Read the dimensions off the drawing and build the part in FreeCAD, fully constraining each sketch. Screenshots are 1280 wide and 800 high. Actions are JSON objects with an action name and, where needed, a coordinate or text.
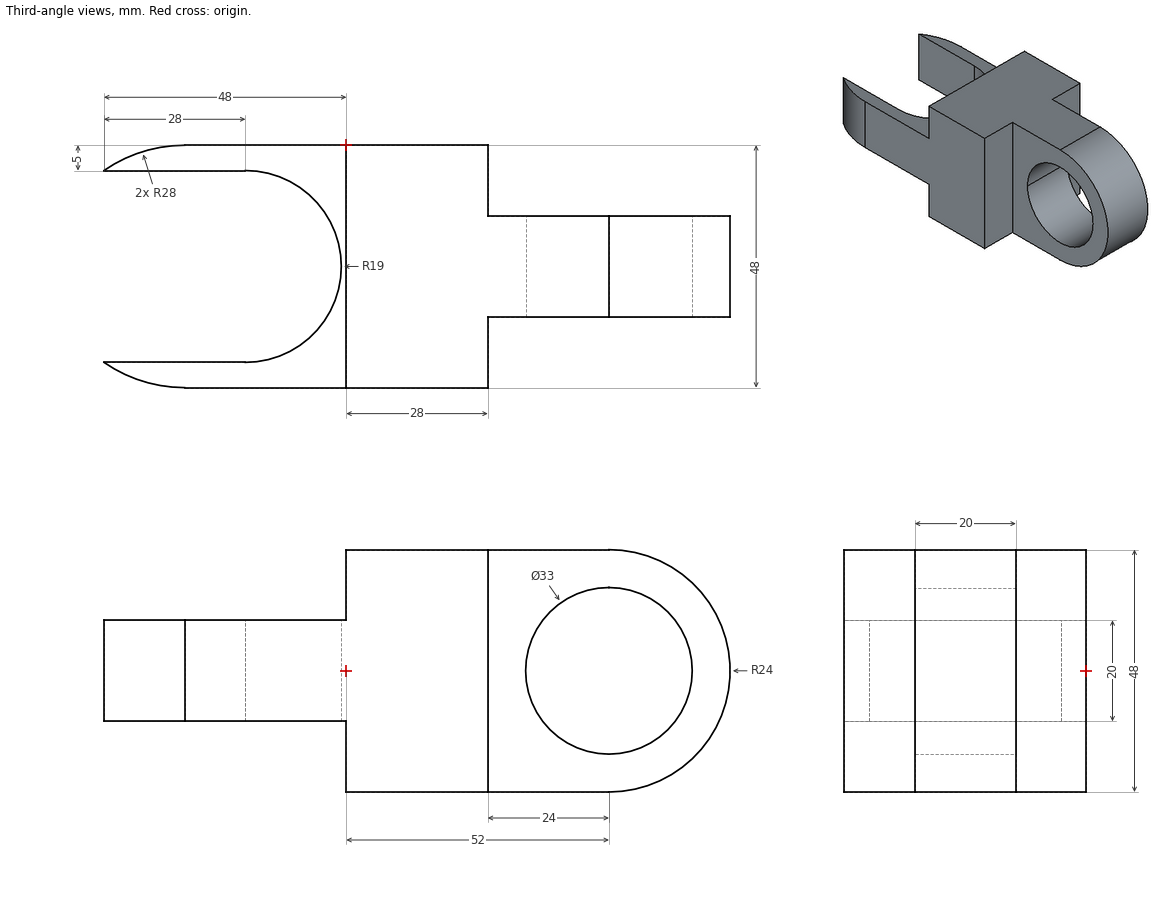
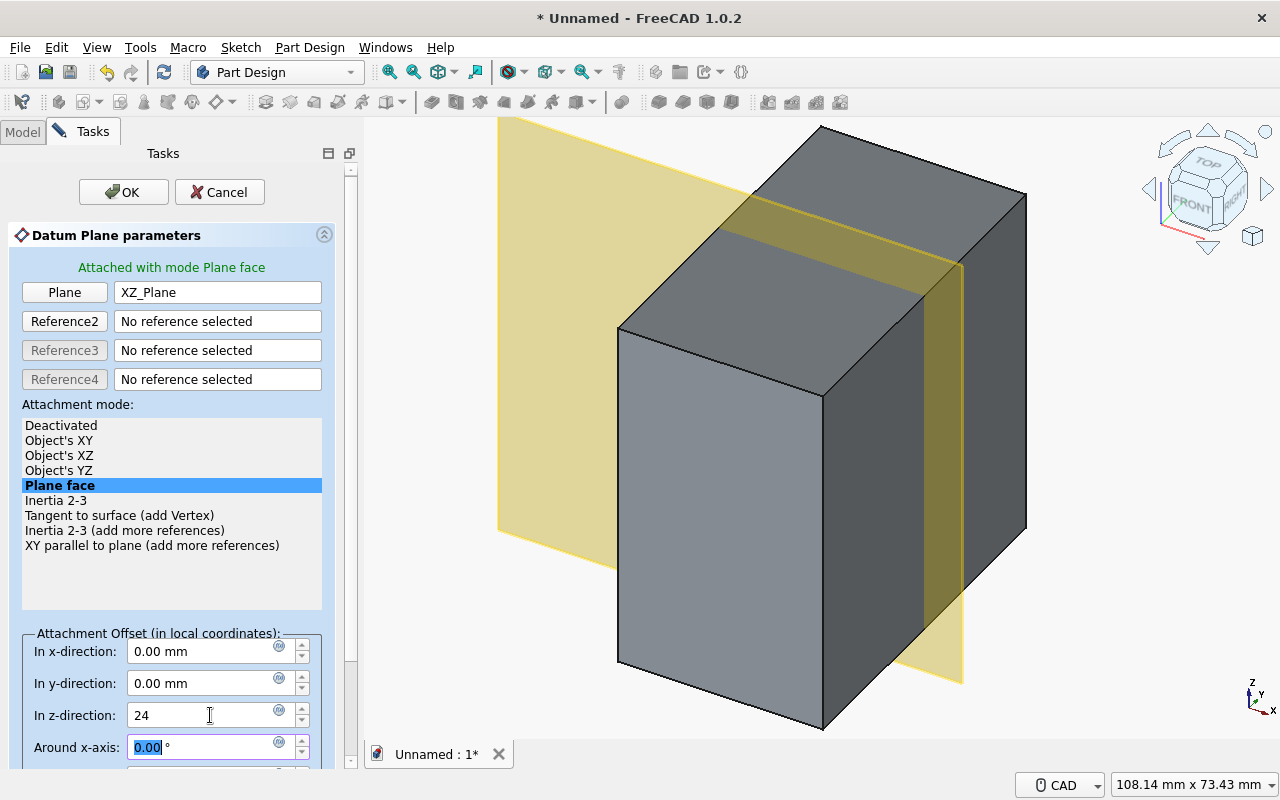
{"action": "left_click", "coordinate": [124, 192]}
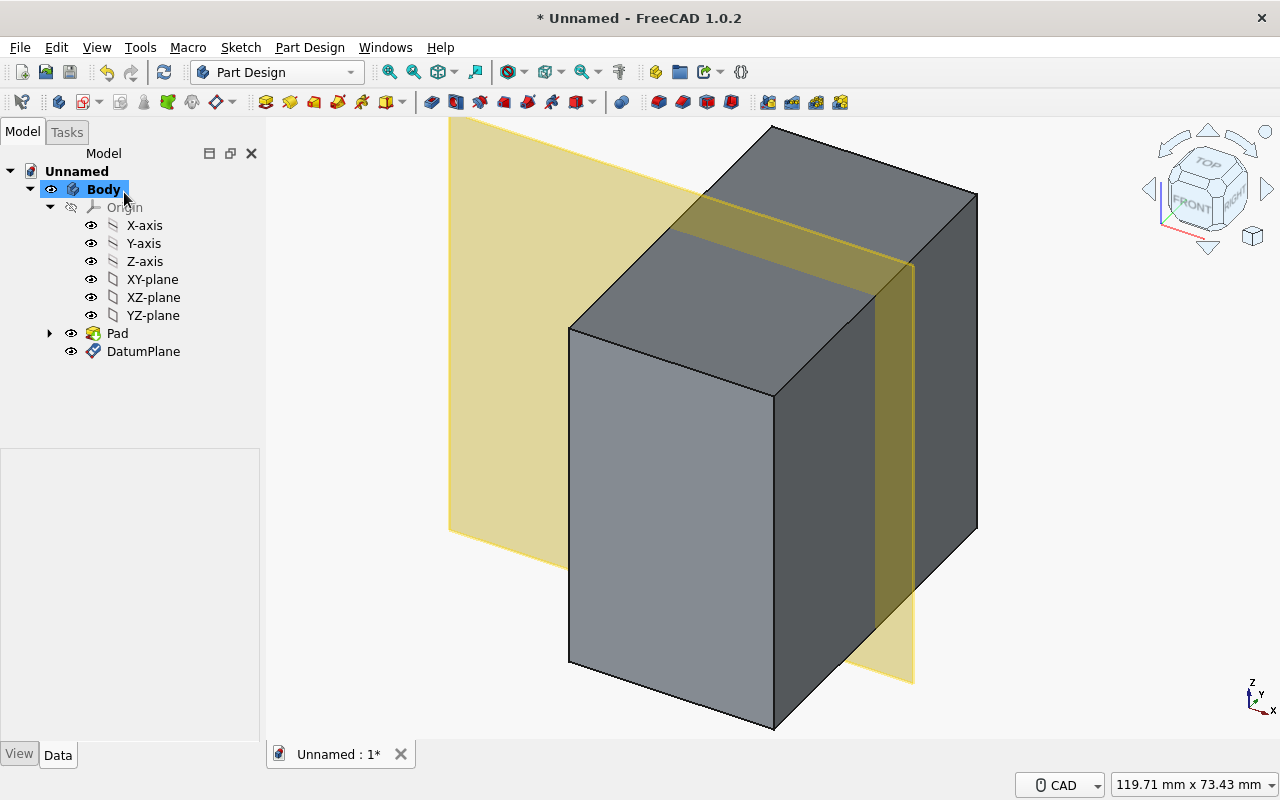
{"action": "left_click", "coordinate": [116, 351]}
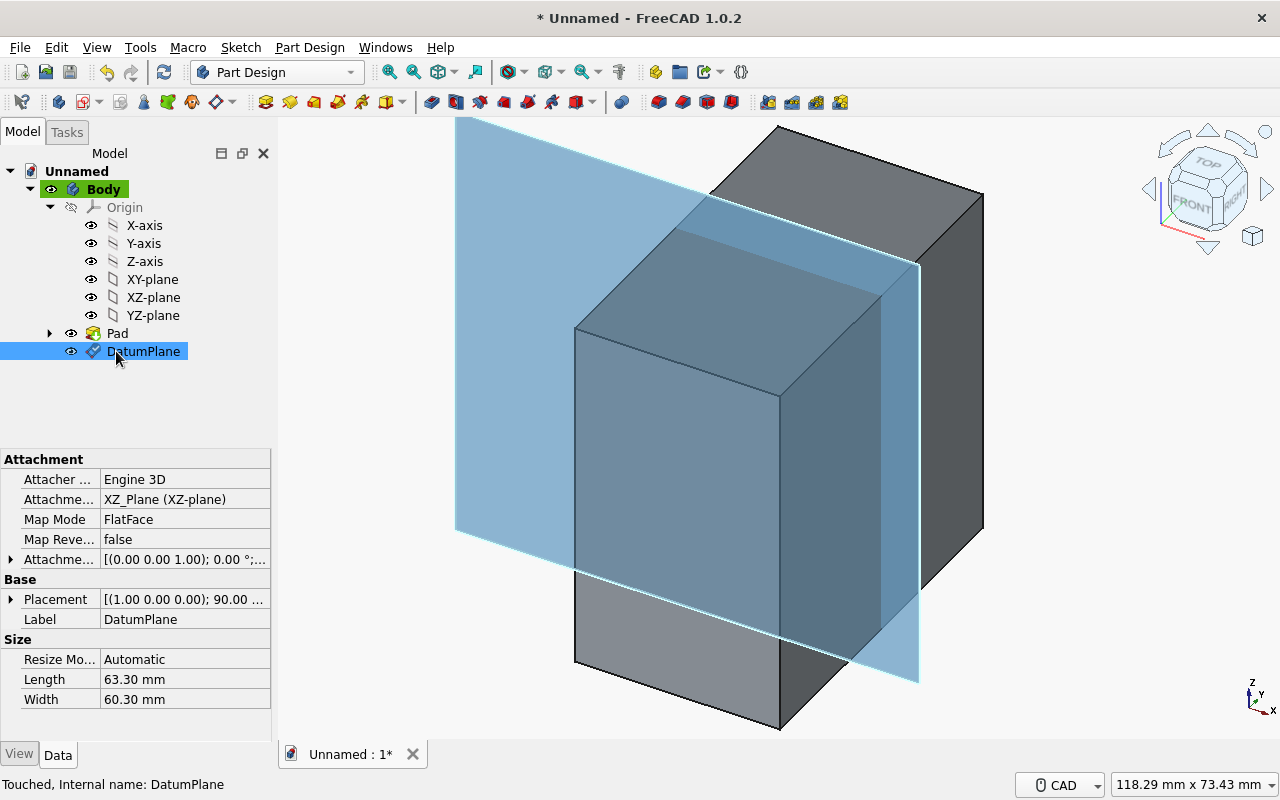
{"action": "left_click", "coordinate": [84, 102]}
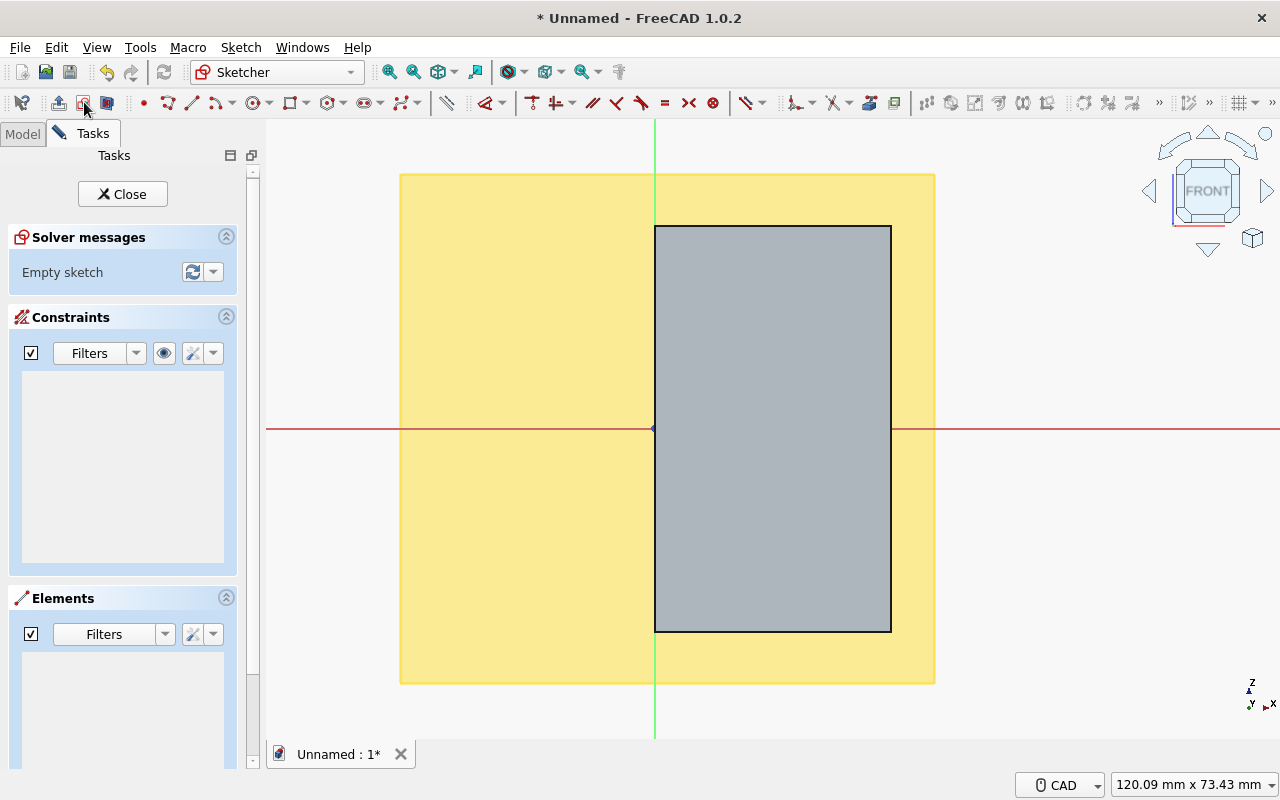
{"action": "left_click", "coordinate": [108, 104]}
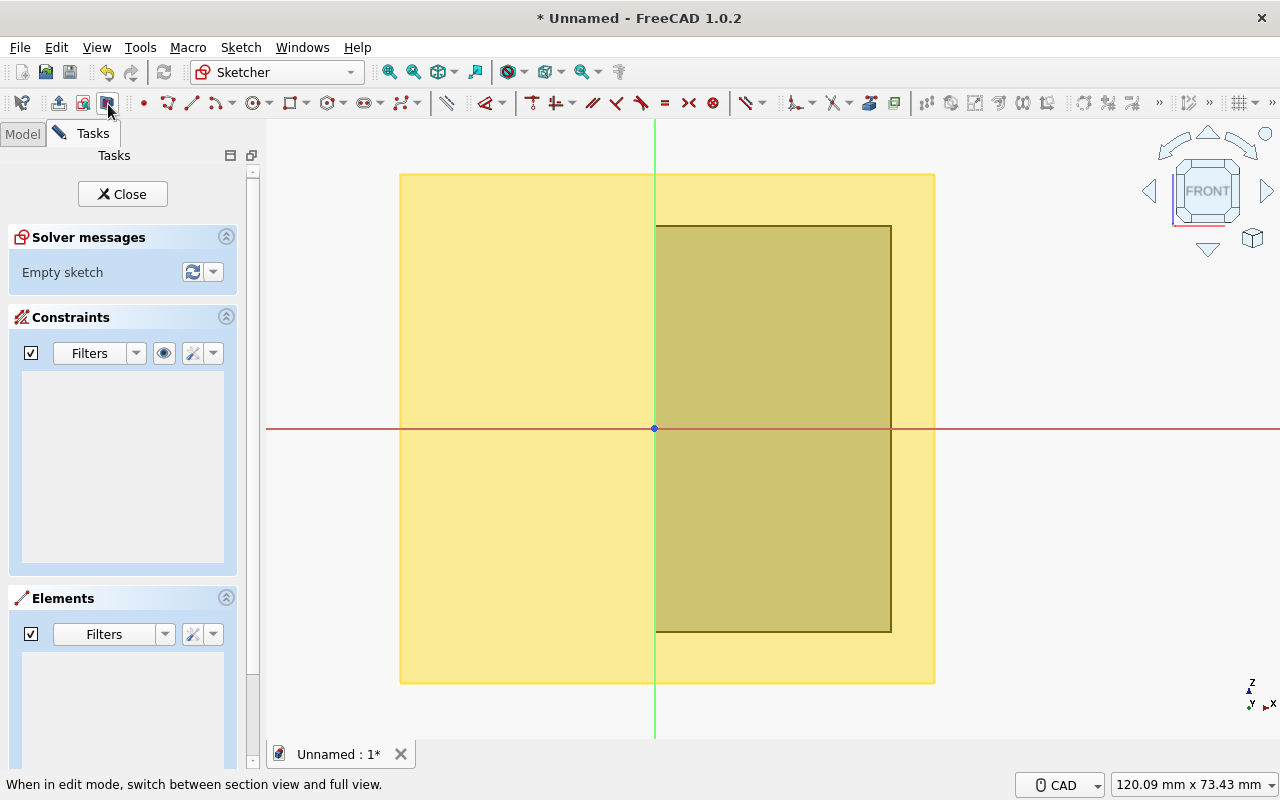
{"action": "scroll", "coordinate": [294, 429], "scroll_direction": "down", "scroll_amount": 2}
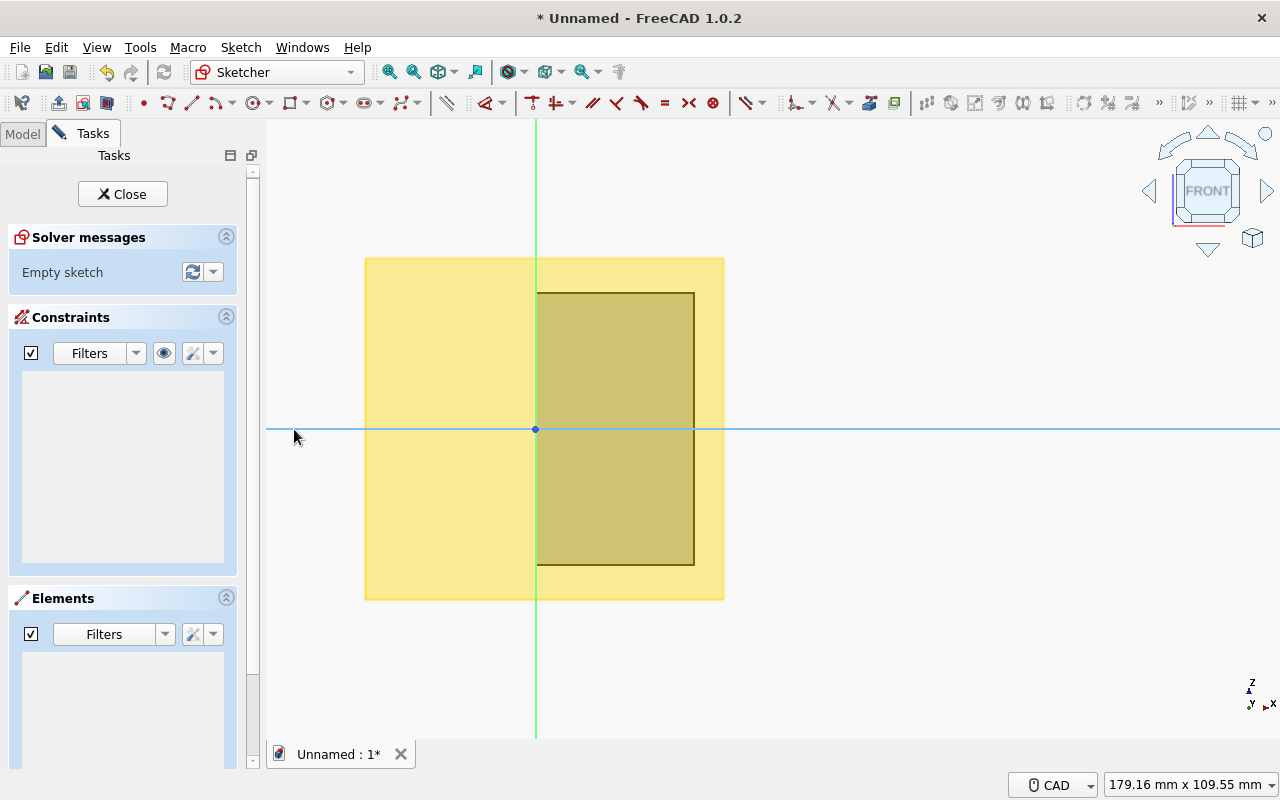
{"action": "key", "text": "g m"}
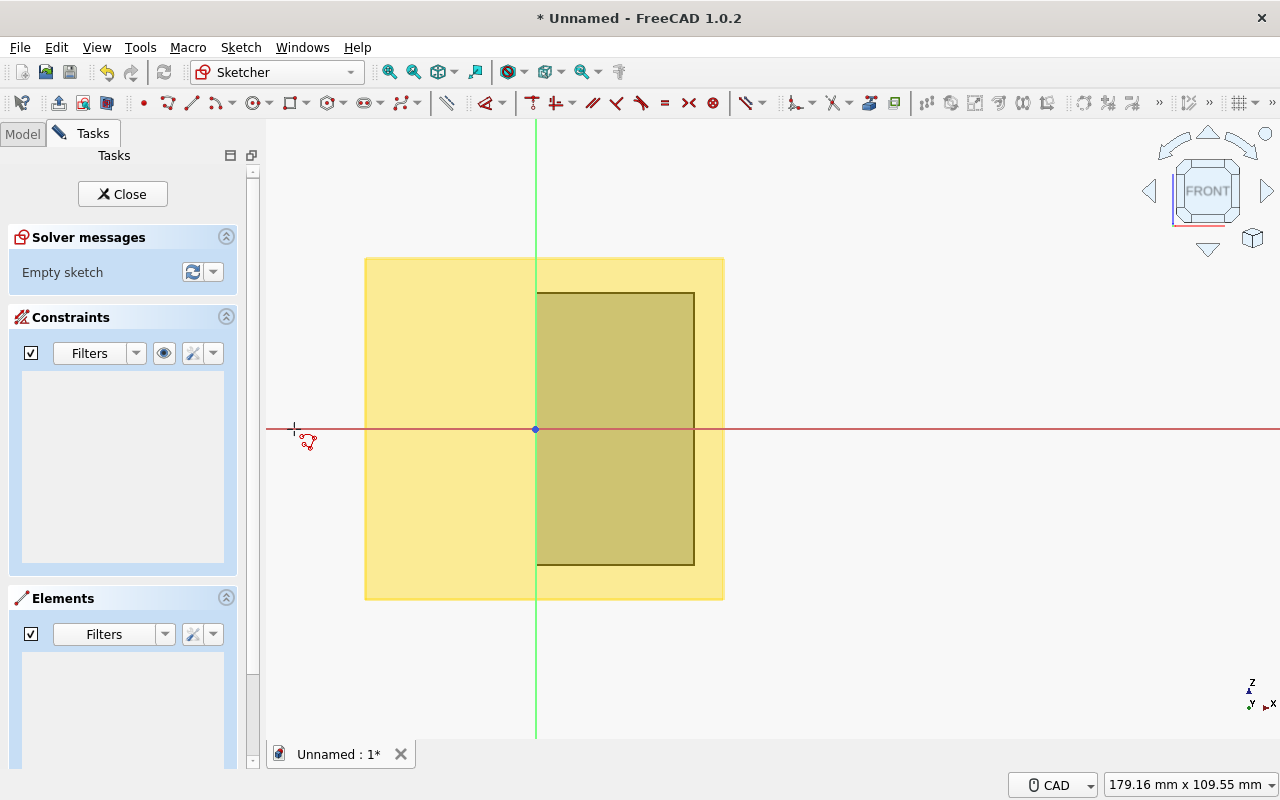
{"action": "left_click", "coordinate": [830, 565]}
{"action": "left_click", "coordinate": [694, 565]}
{"action": "left_click", "coordinate": [694, 293]}
{"action": "left_click", "coordinate": [830, 293]}
{"action": "right_click", "coordinate": [830, 293]}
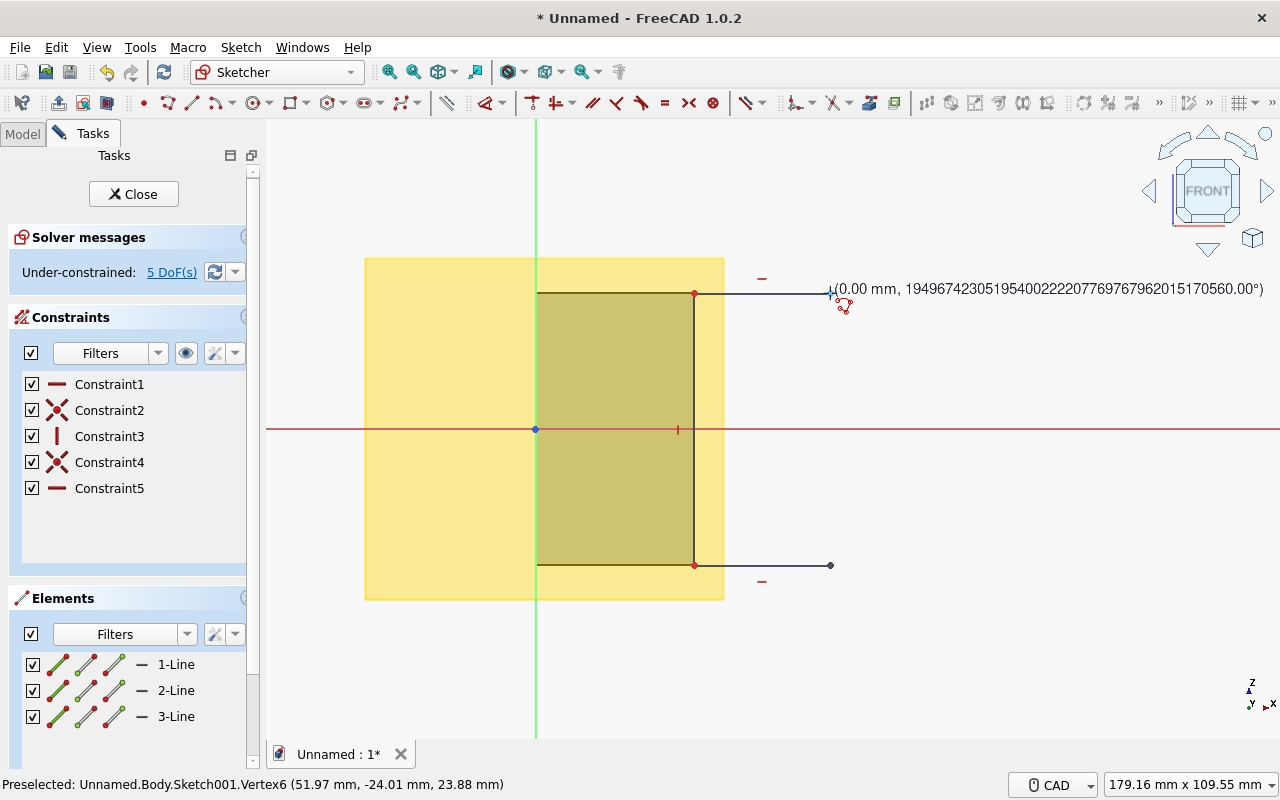
{"action": "left_click", "coordinate": [234, 104]}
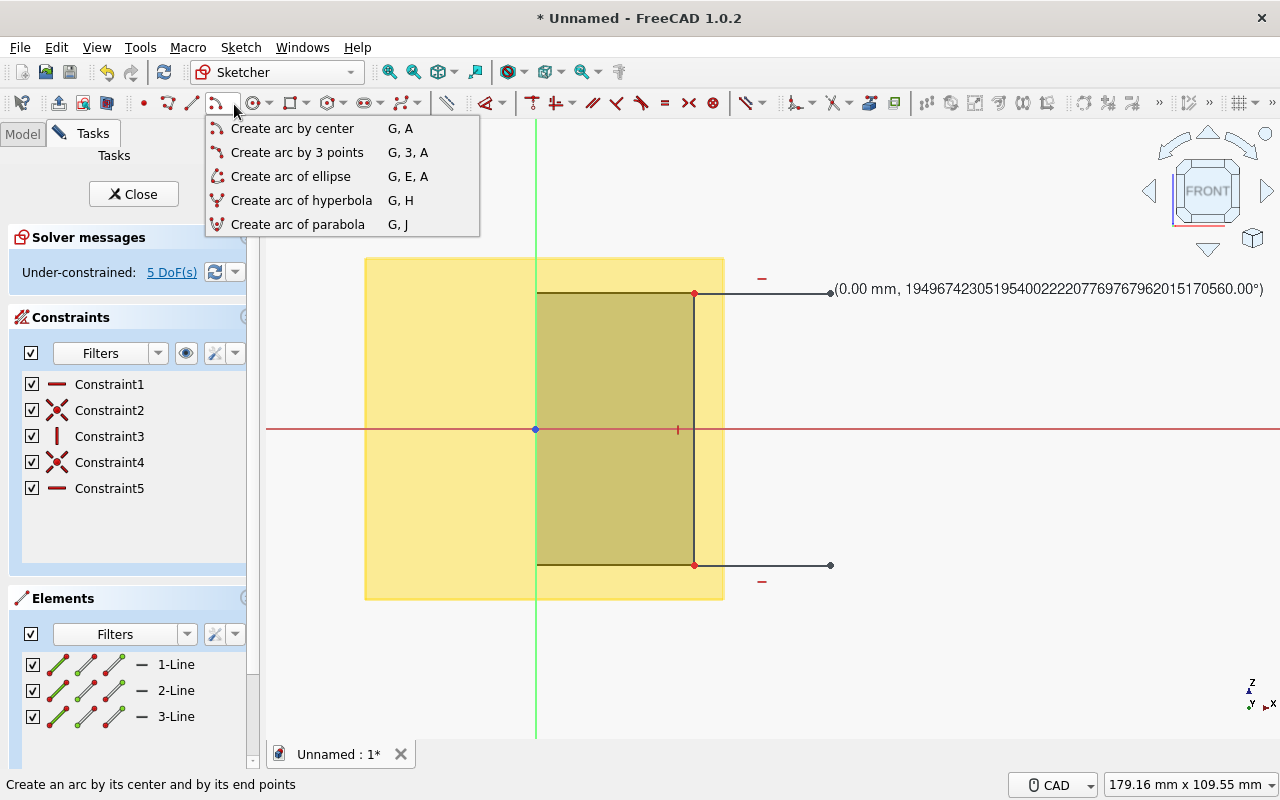
{"action": "left_click", "coordinate": [342, 152]}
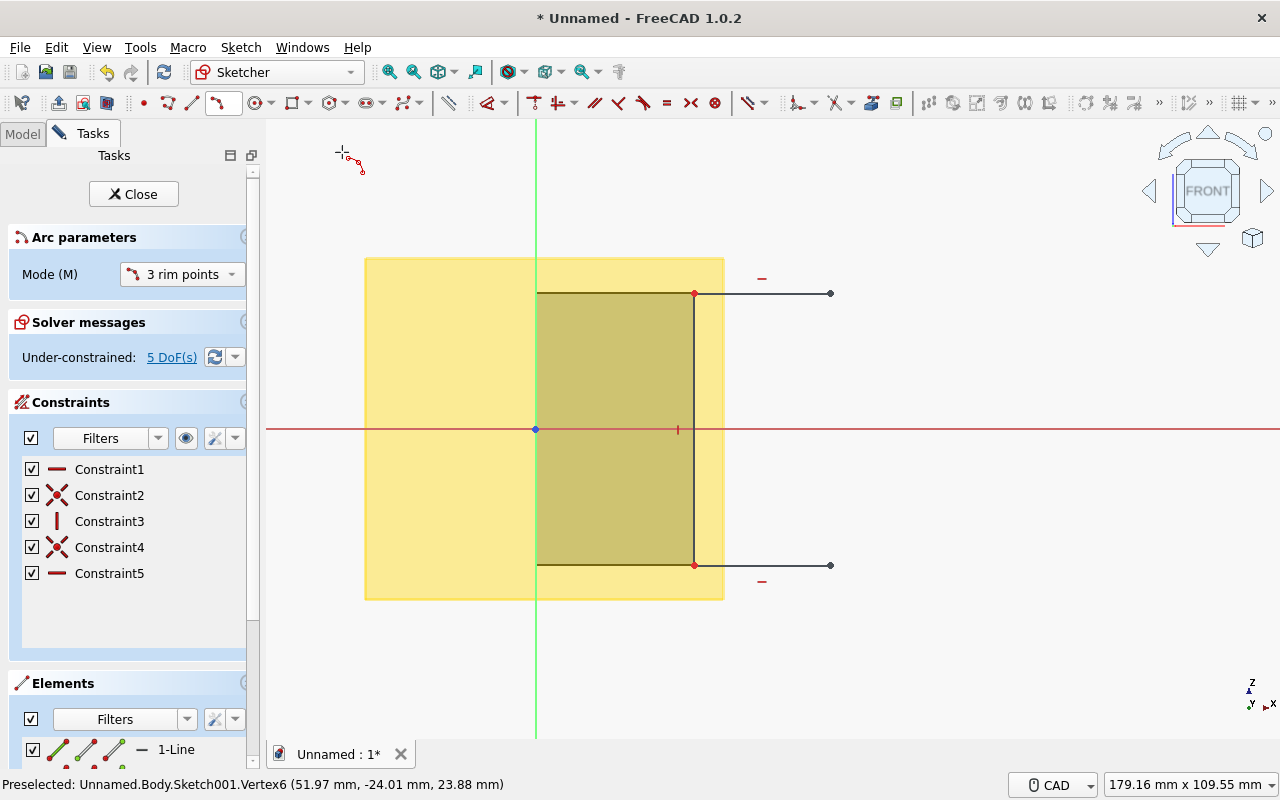
{"action": "left_click", "coordinate": [830, 294]}
{"action": "left_click", "coordinate": [830, 566]}
{"action": "left_click", "coordinate": [959, 471]}
{"action": "key", "text": "Escape"}